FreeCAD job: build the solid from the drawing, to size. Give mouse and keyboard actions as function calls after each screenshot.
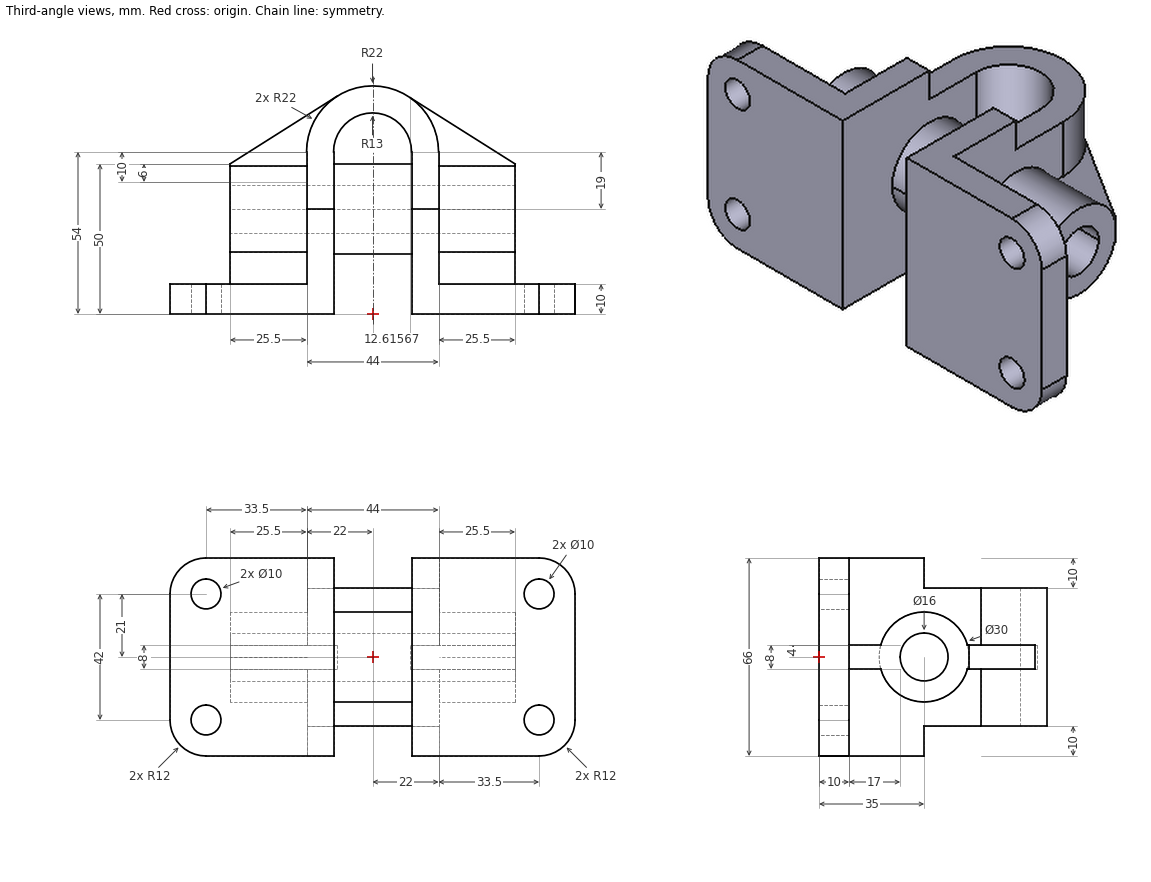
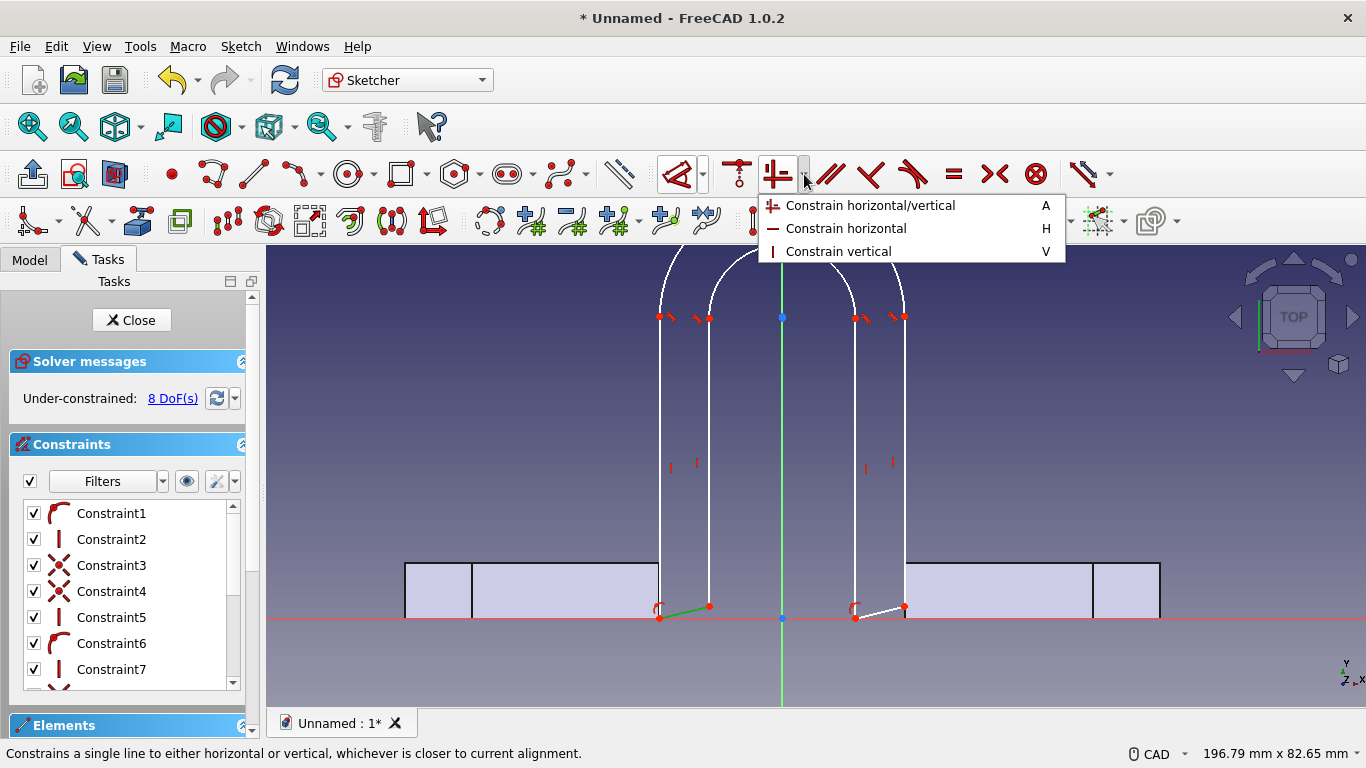
click(912, 228)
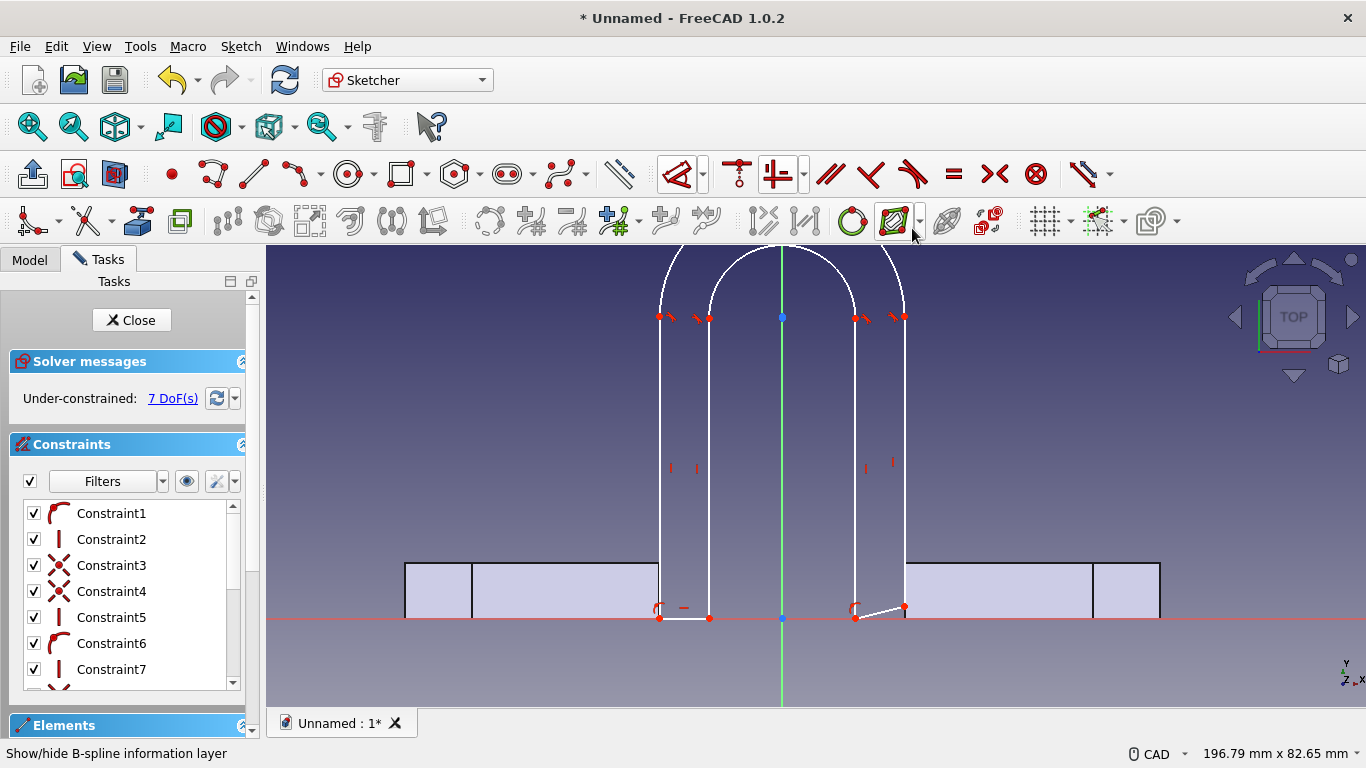
click(870, 615)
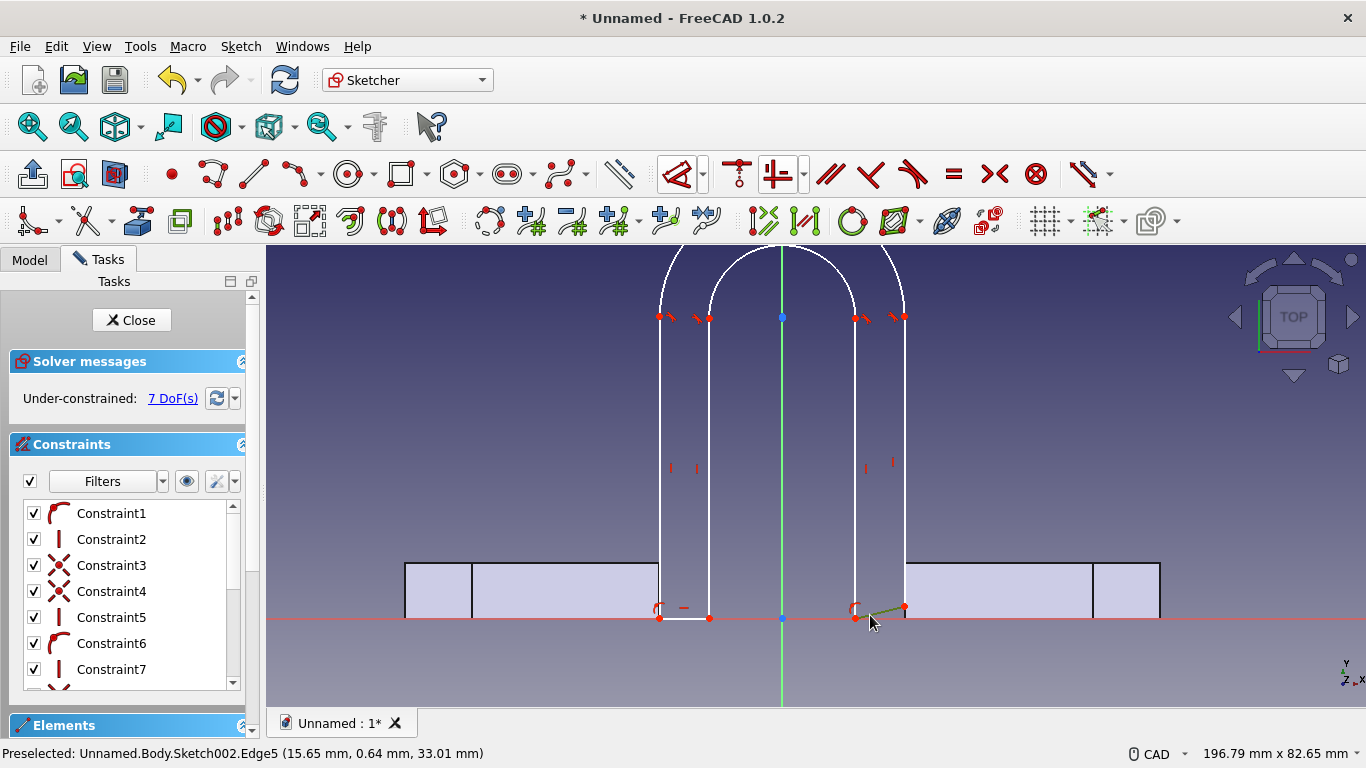
key(h)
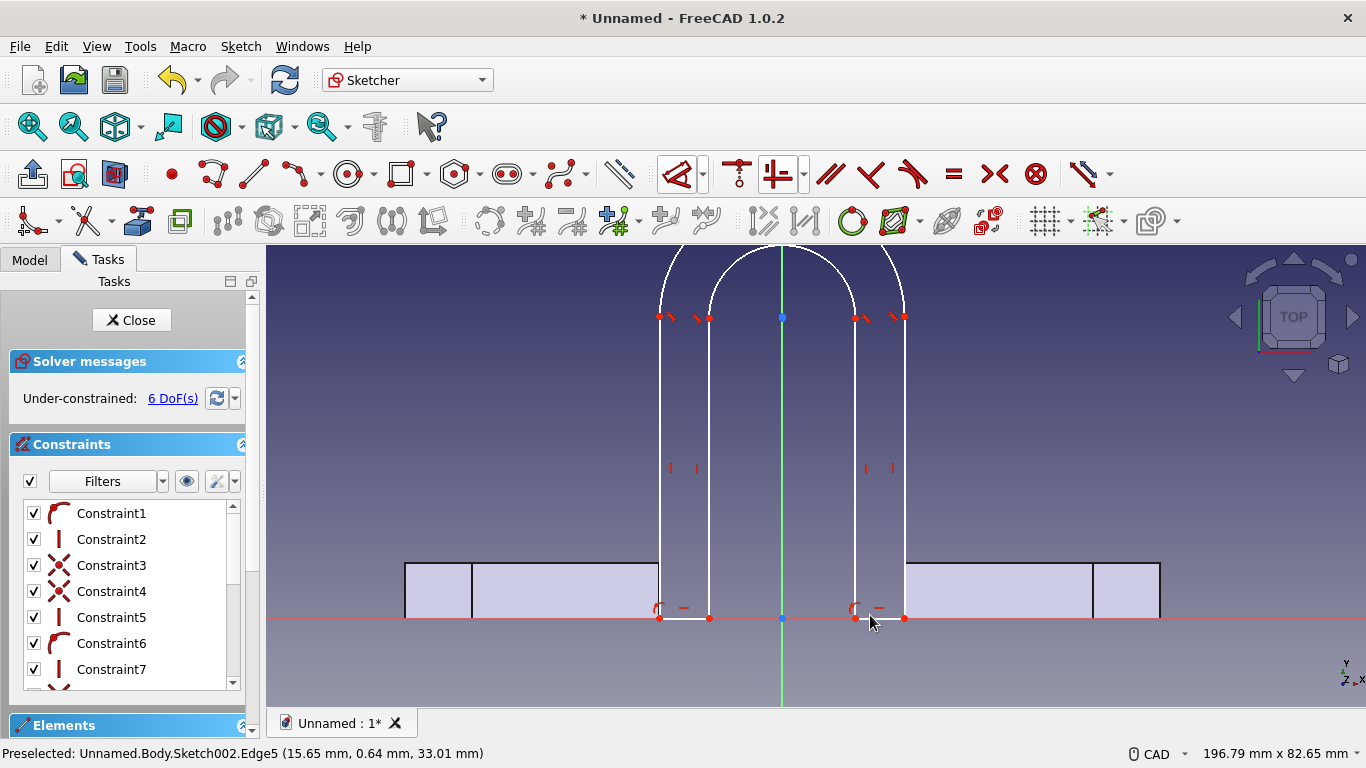
click(841, 275)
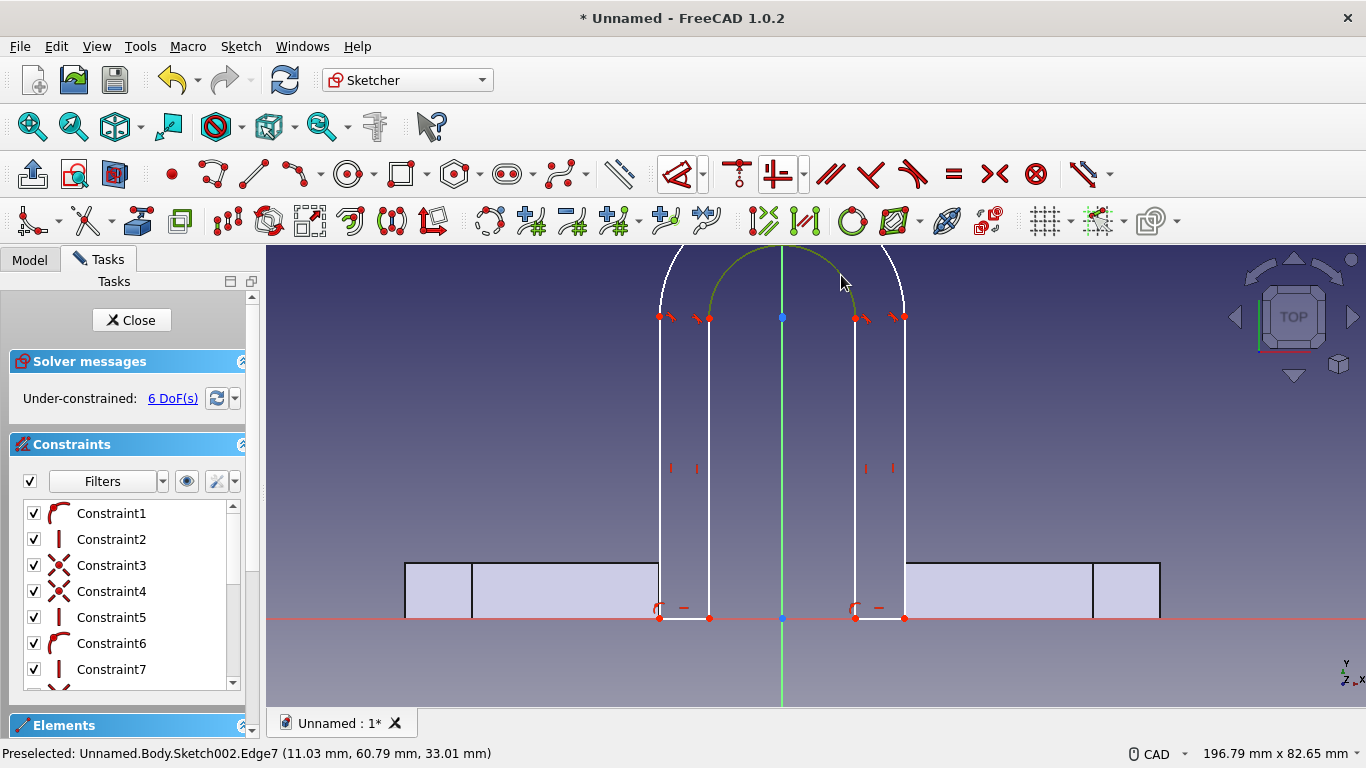
scroll(677, 618, down, 2)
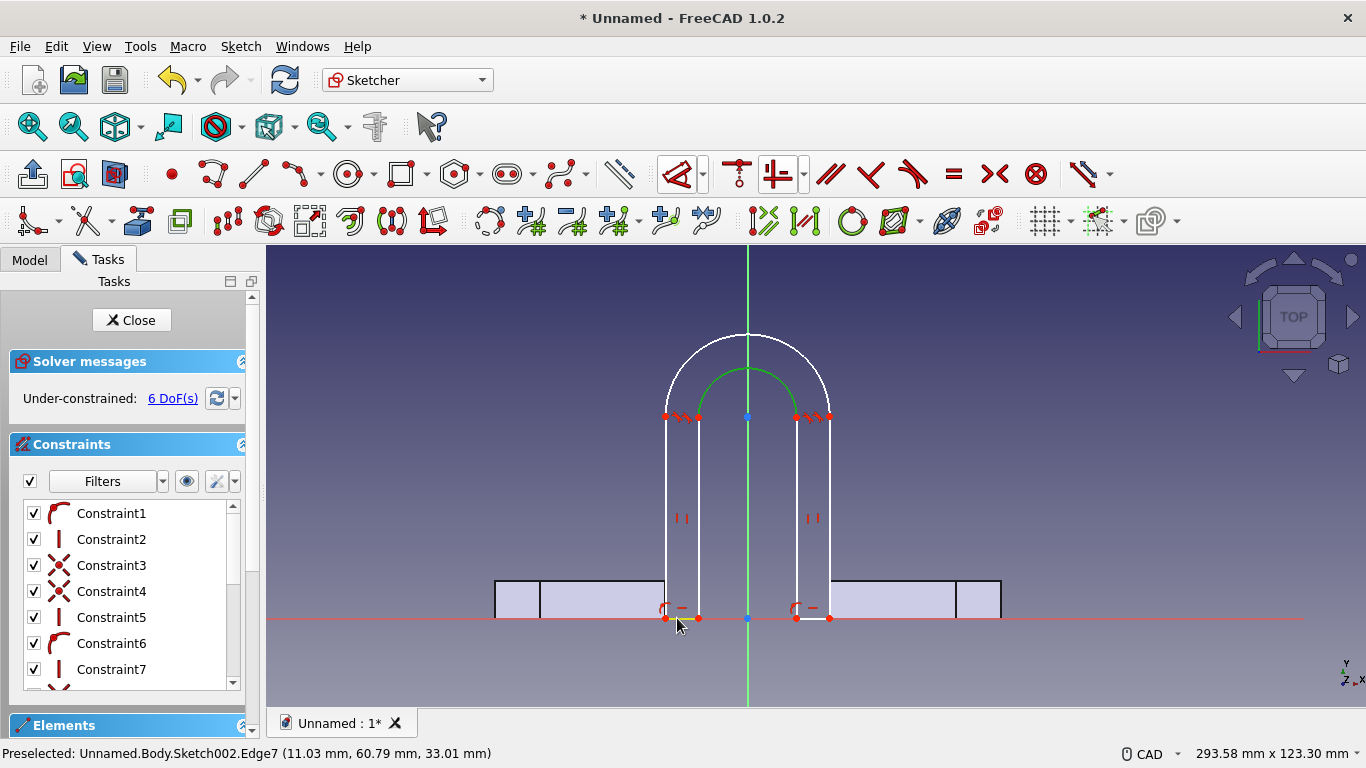
click(796, 350)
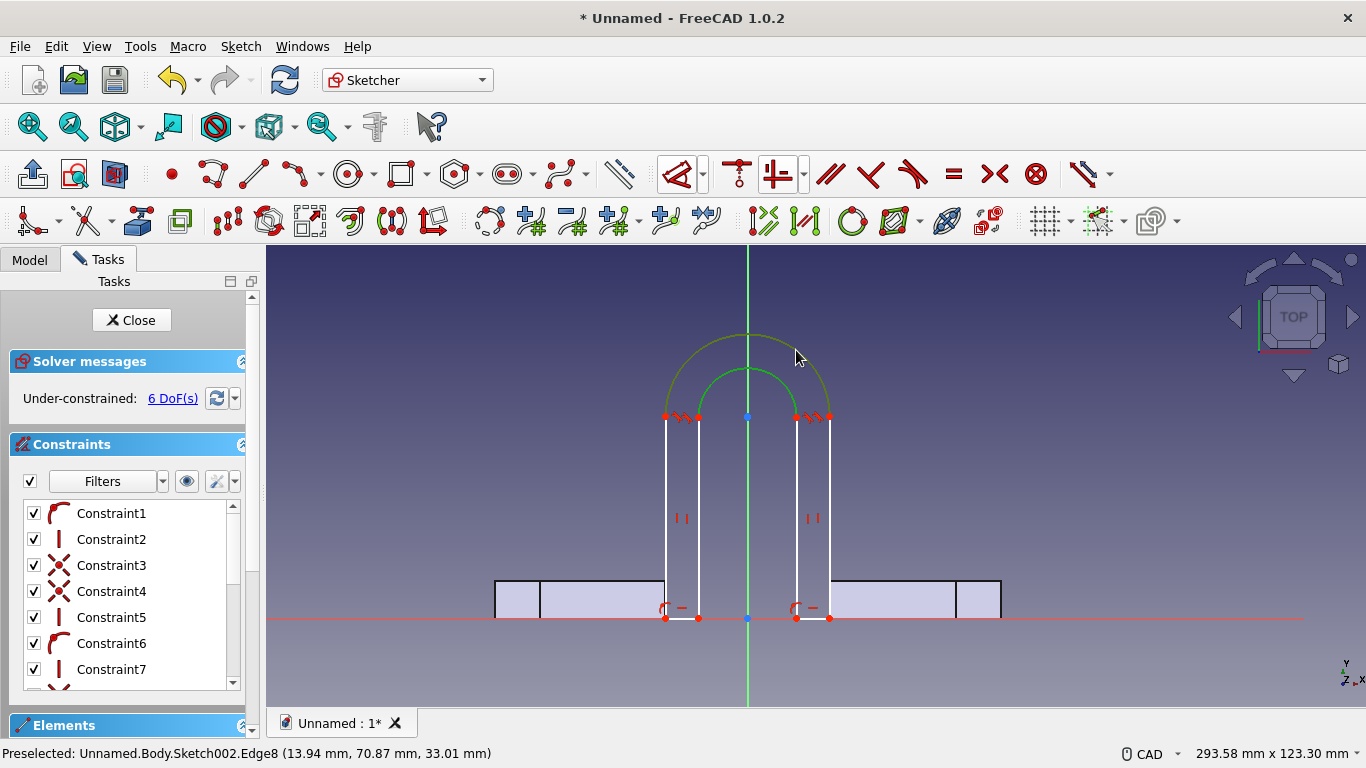
click(737, 174)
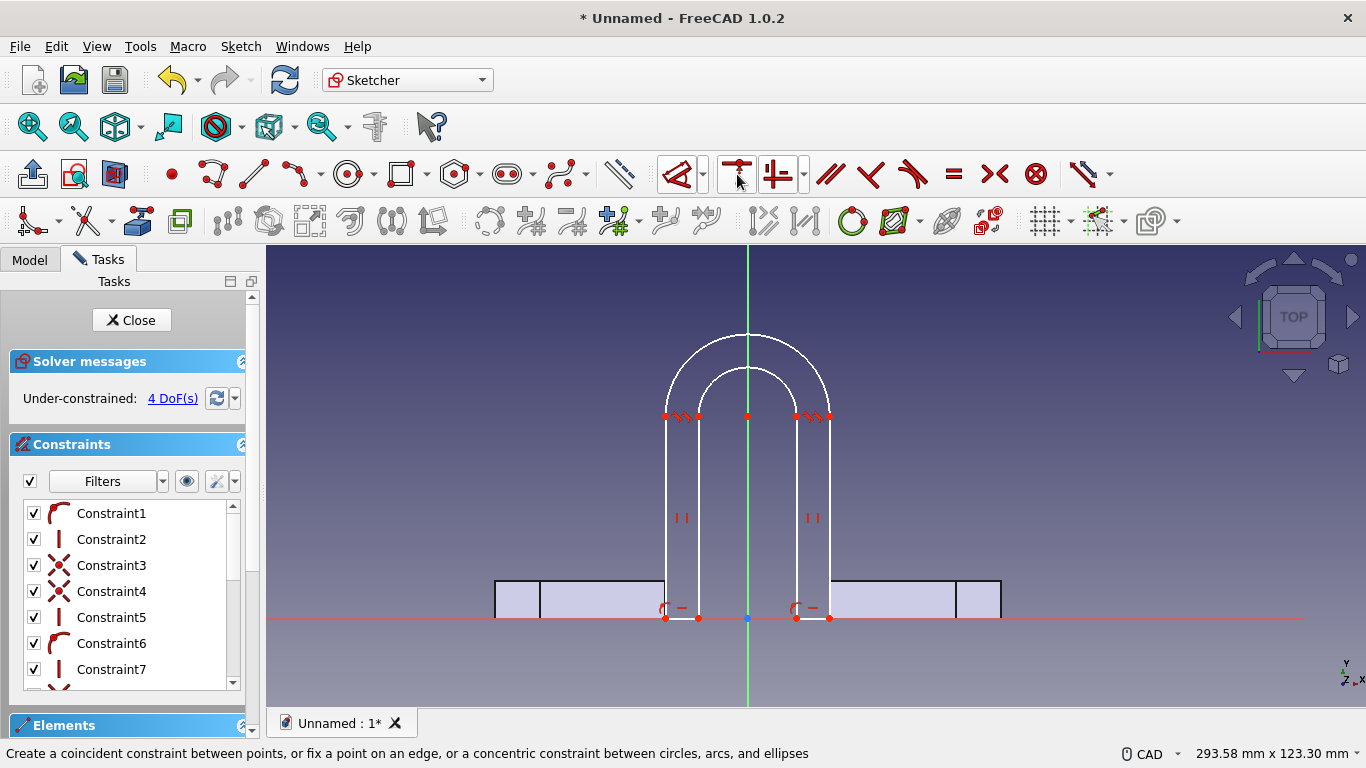
click(748, 416)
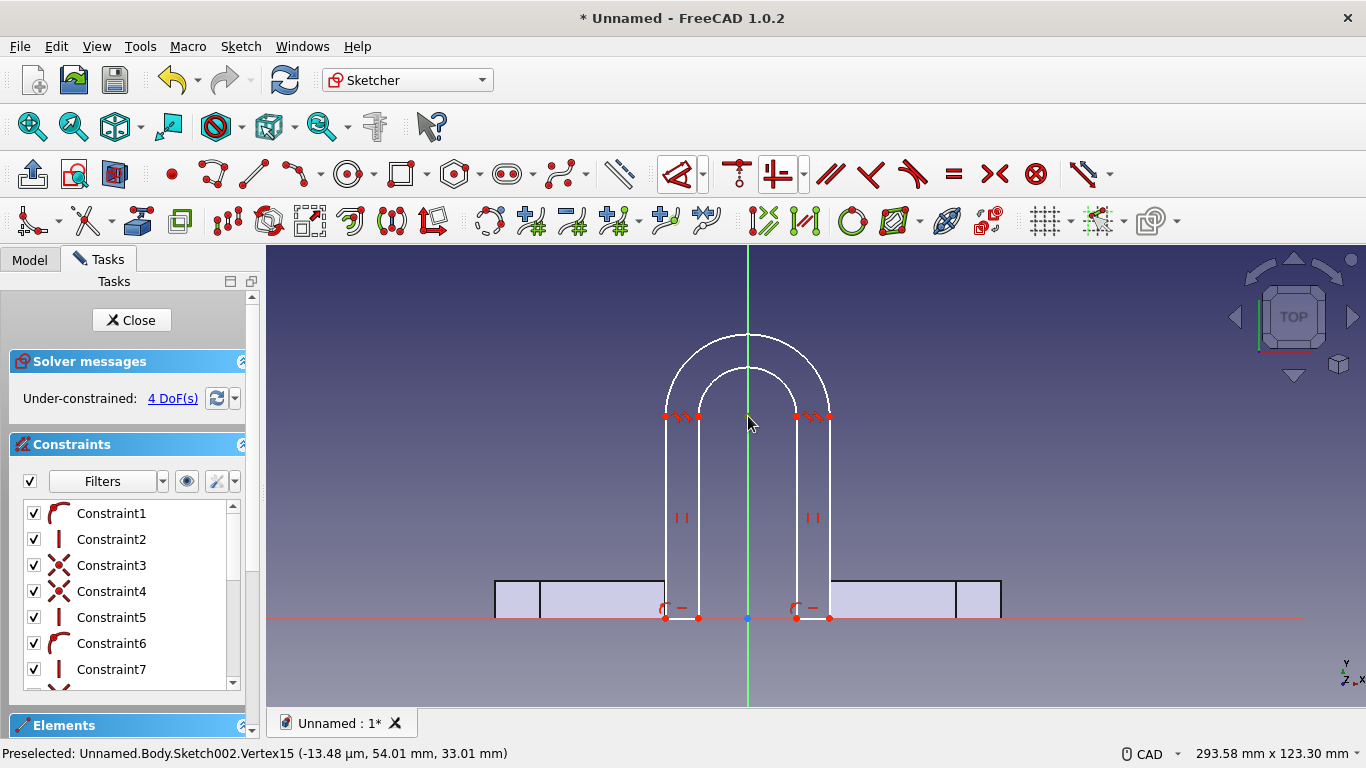
click(748, 650)